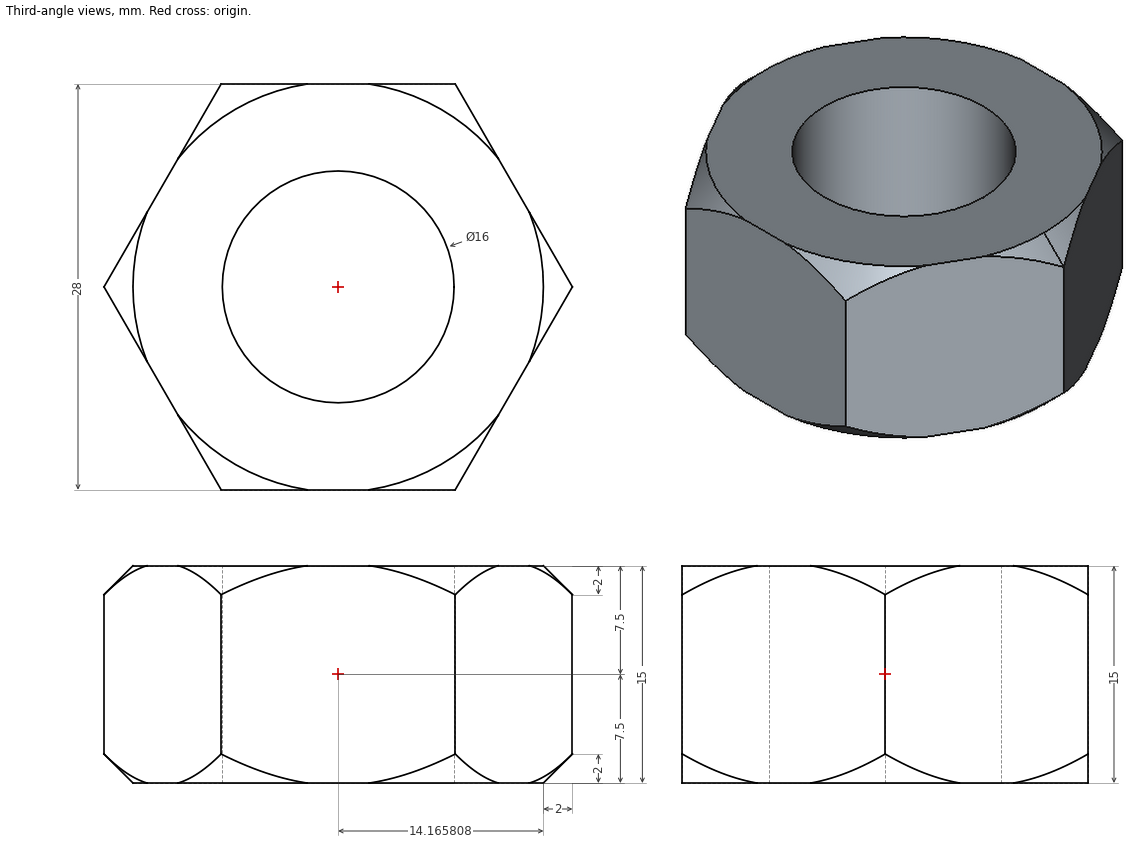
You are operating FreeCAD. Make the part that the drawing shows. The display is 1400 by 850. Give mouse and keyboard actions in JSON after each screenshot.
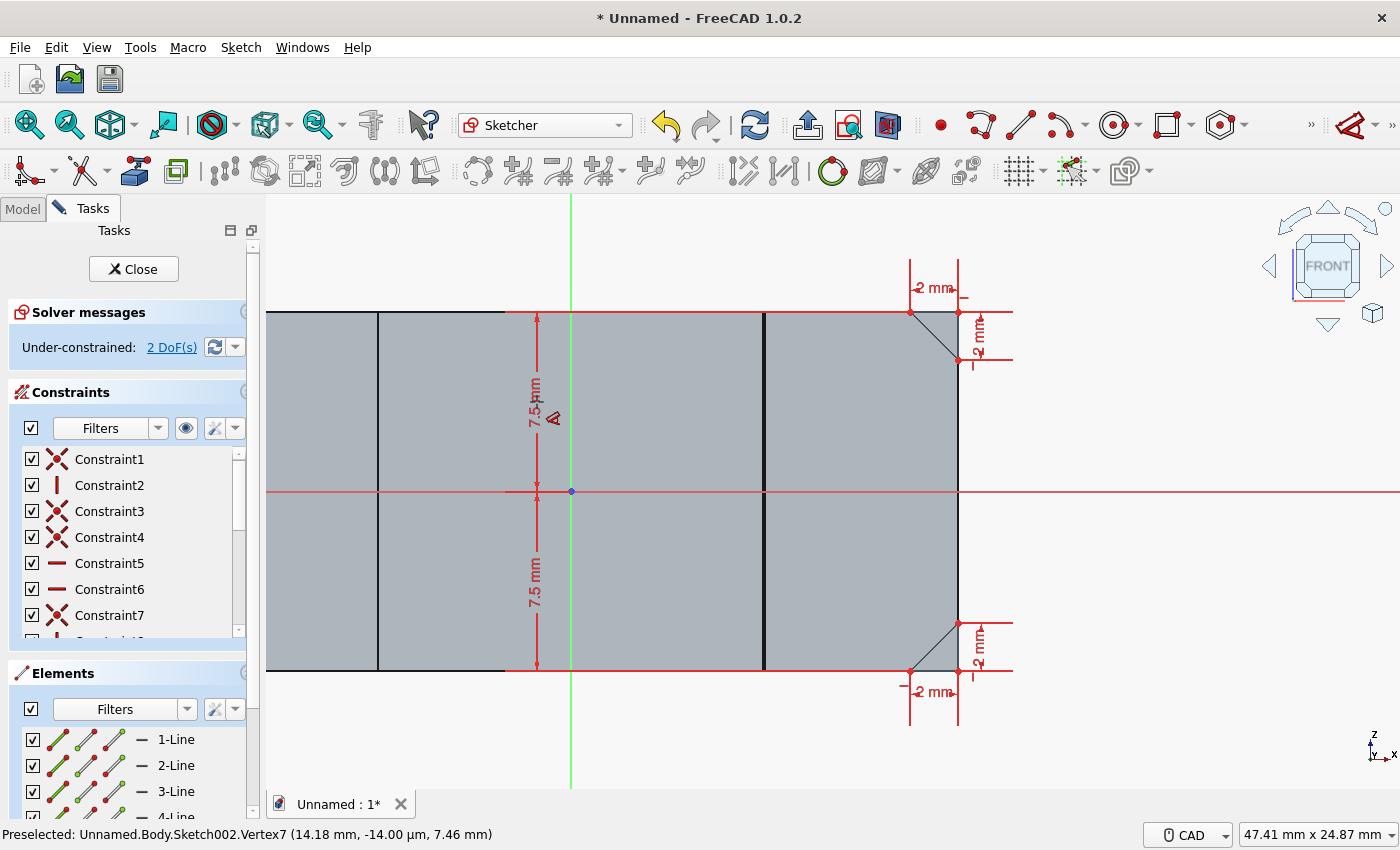
{"action": "left_click", "coordinate": [910, 671]}
{"action": "left_click", "coordinate": [741, 705]}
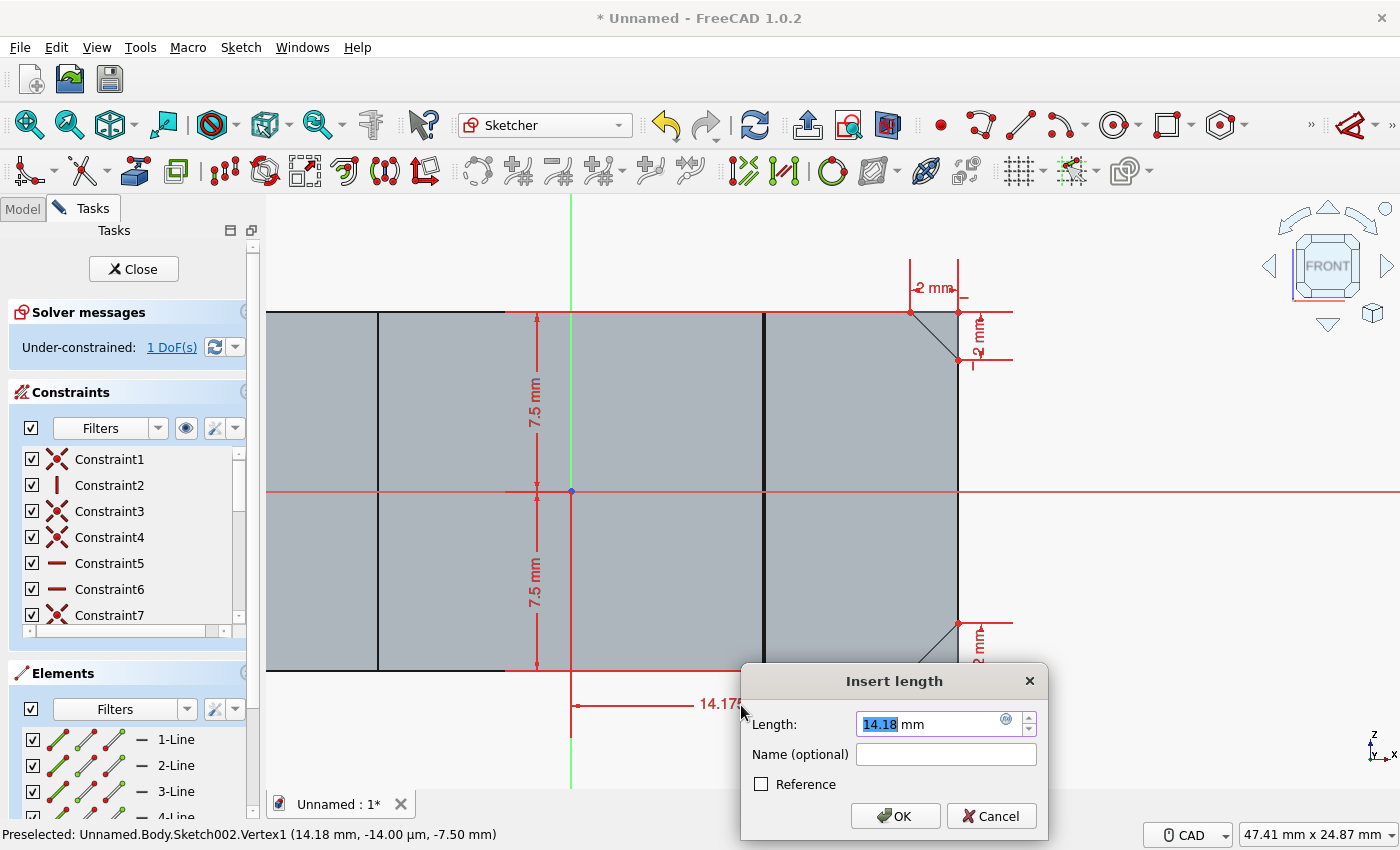
{"action": "type", "text": "14.165808"}
{"action": "key", "text": "Return"}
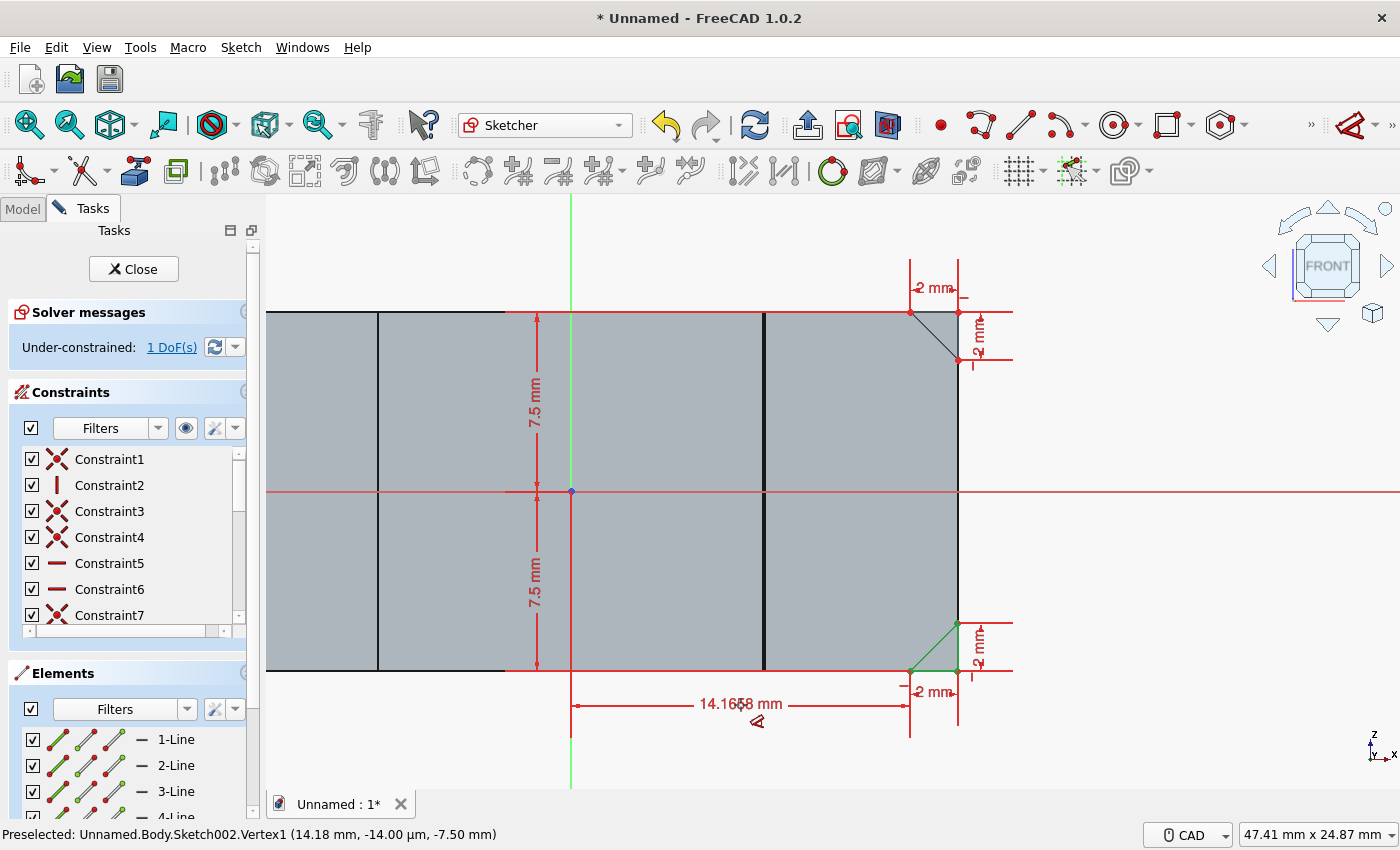
{"action": "left_click", "coordinate": [910, 312]}
{"action": "left_click", "coordinate": [741, 278]}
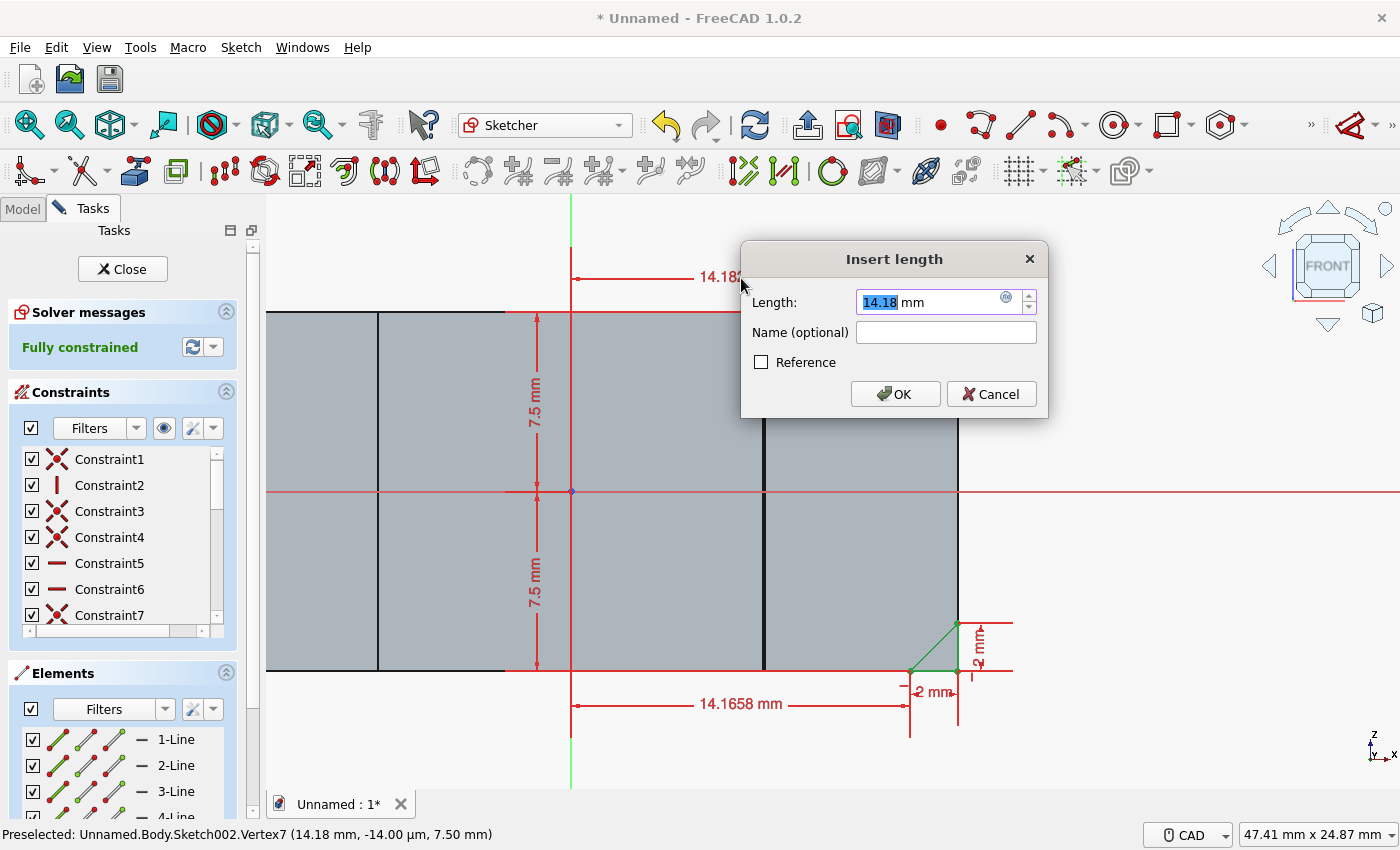
{"action": "type", "text": "14.165808"}
{"action": "key", "text": "Return"}
{"action": "key", "text": "Escape"}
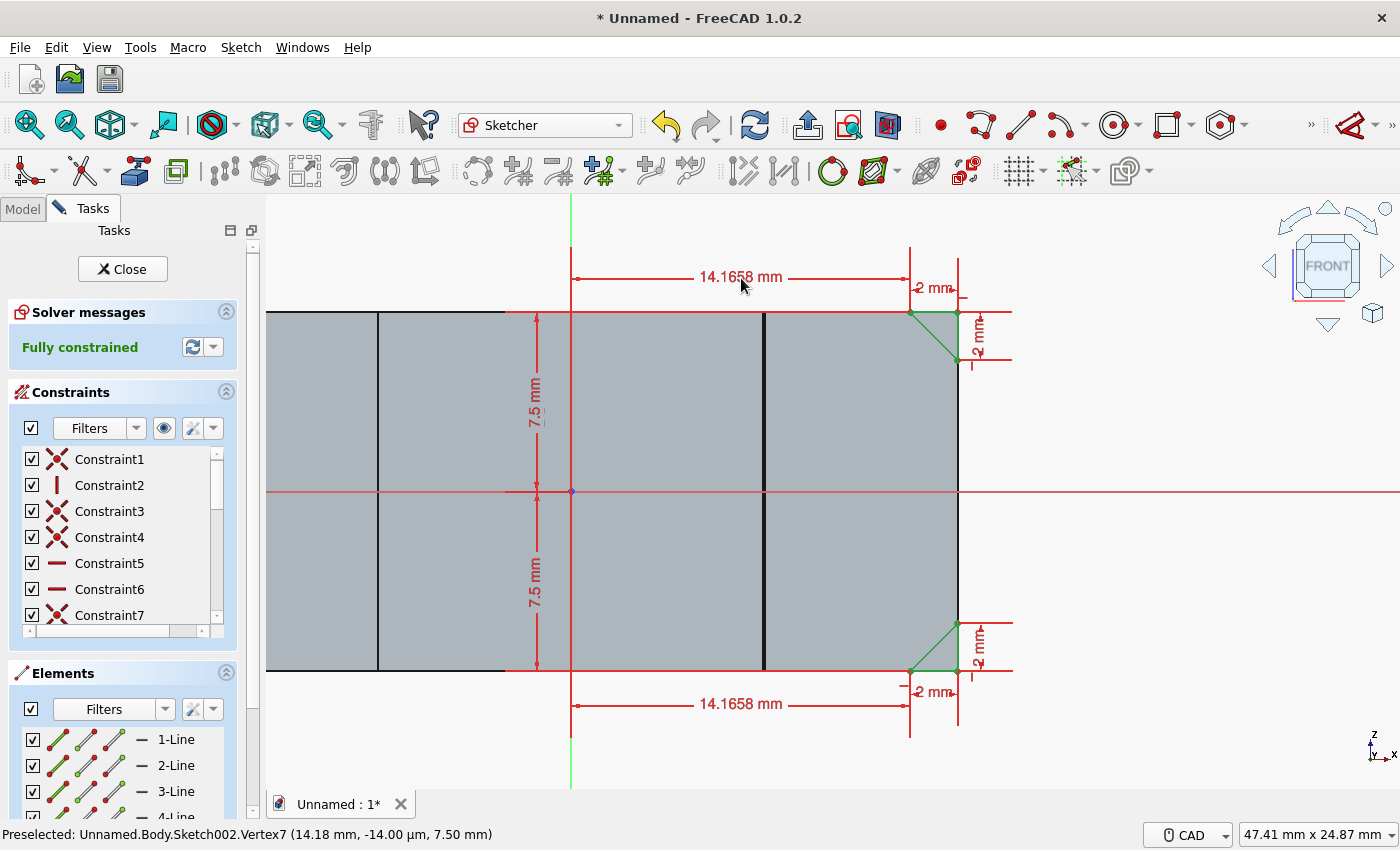
{"action": "left_click", "coordinate": [123, 269]}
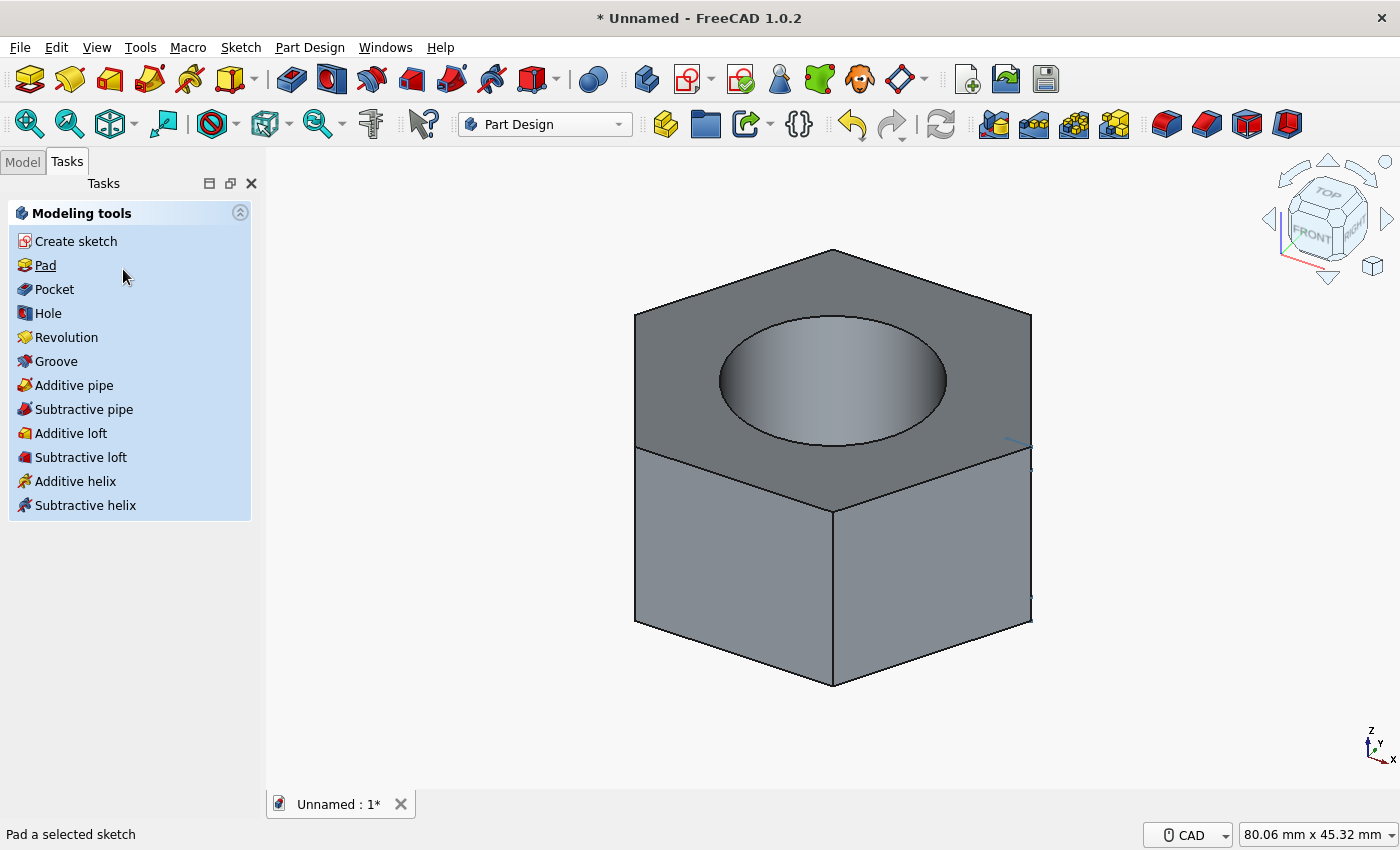
{"action": "left_click", "coordinate": [372, 80]}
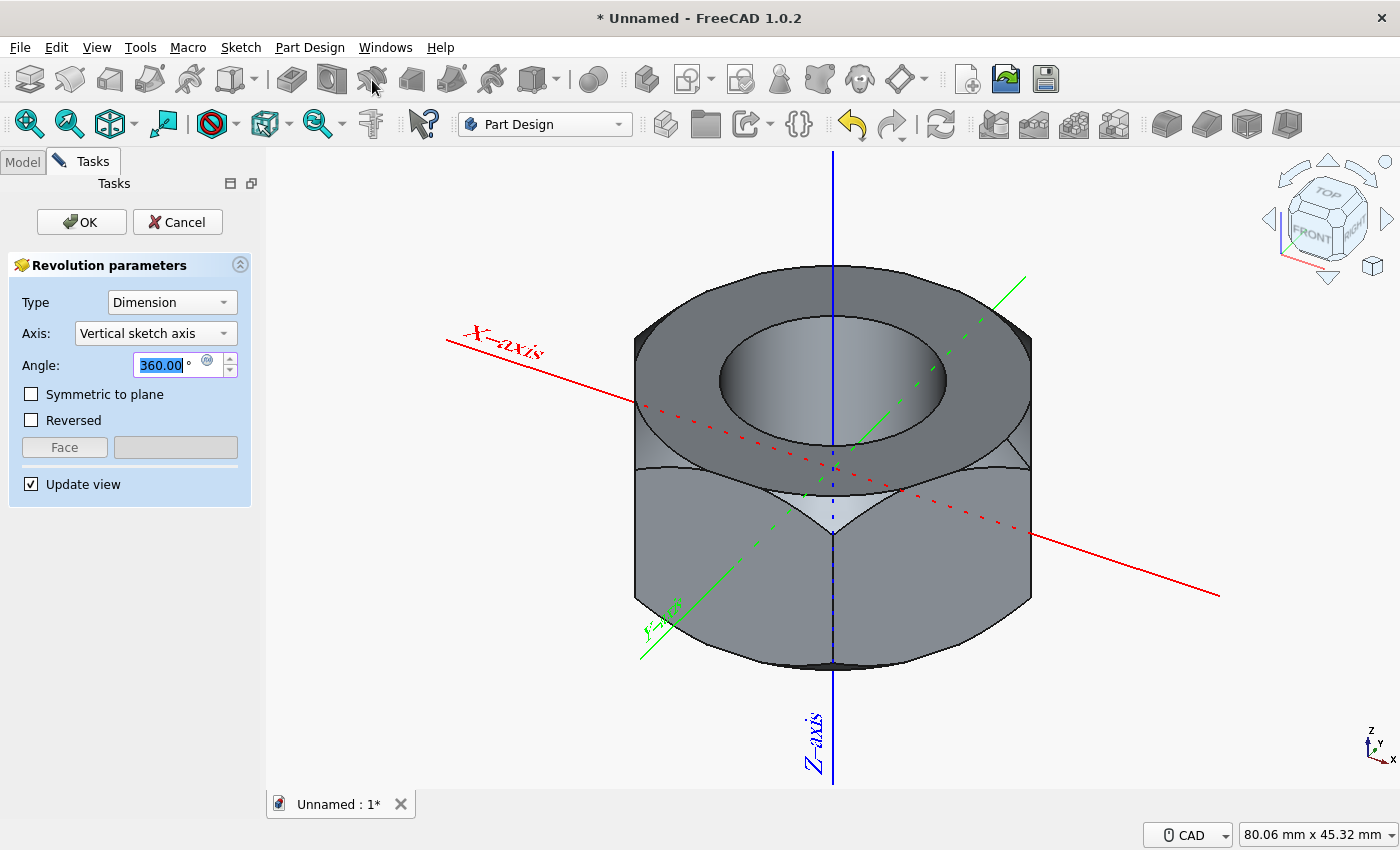
{"action": "left_click", "coordinate": [82, 222]}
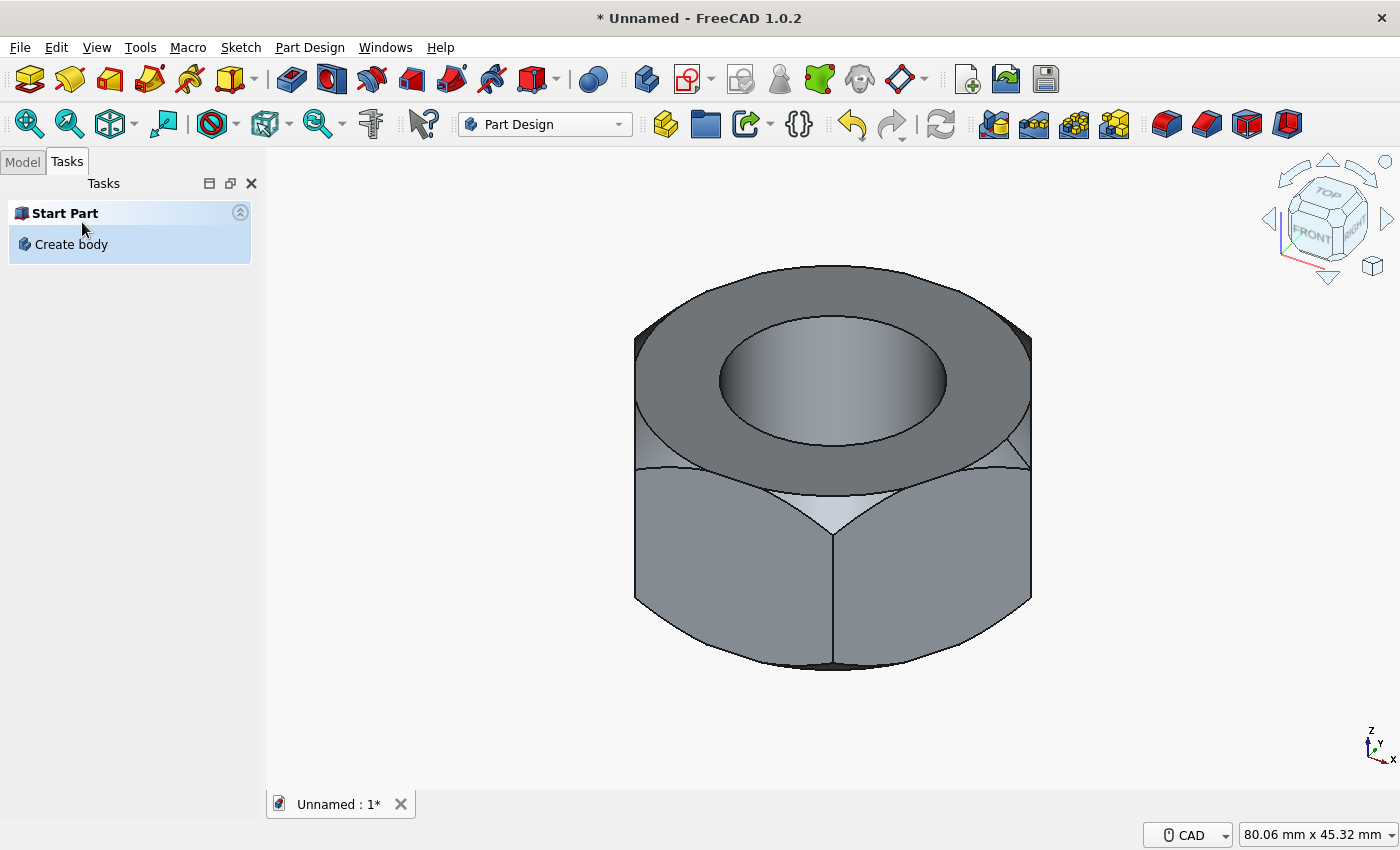
{"action": "key", "text": "0"}